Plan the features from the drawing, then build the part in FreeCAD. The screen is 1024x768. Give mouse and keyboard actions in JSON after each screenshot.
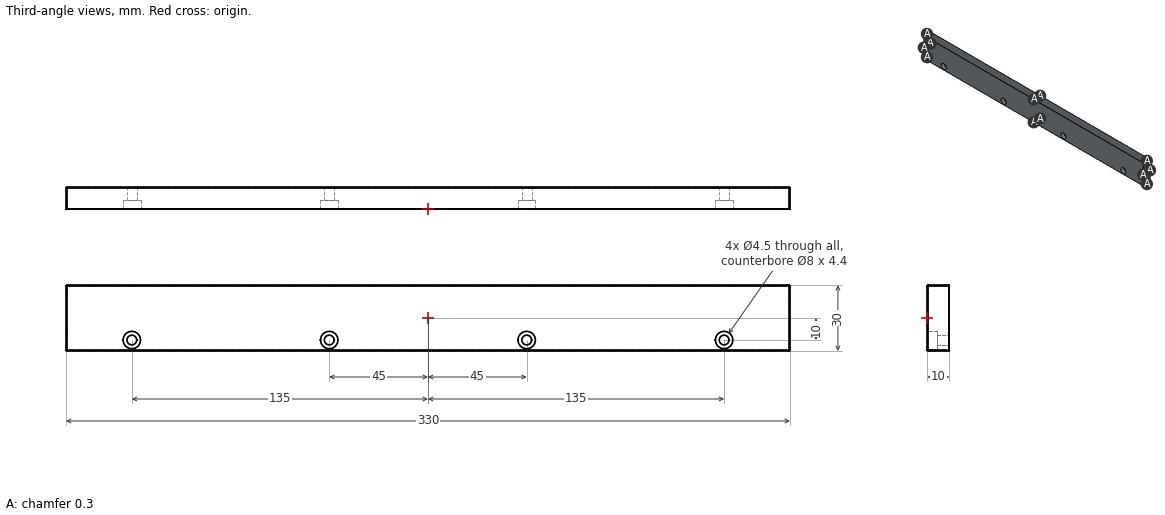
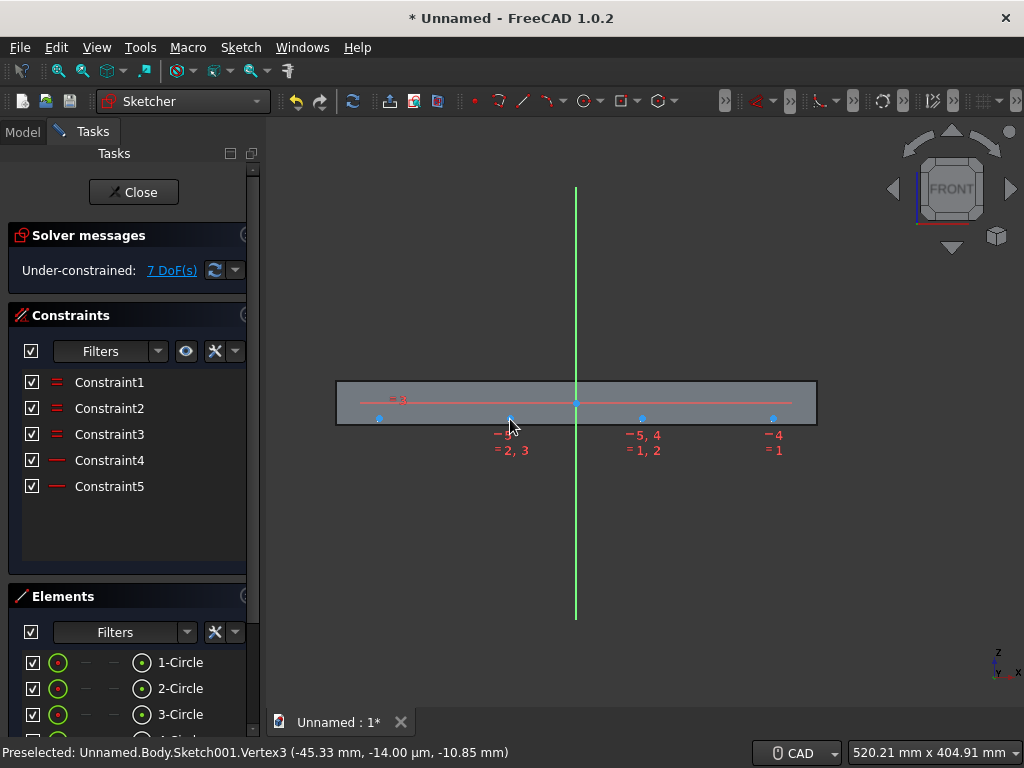
{"action": "left_click", "coordinate": [510, 419]}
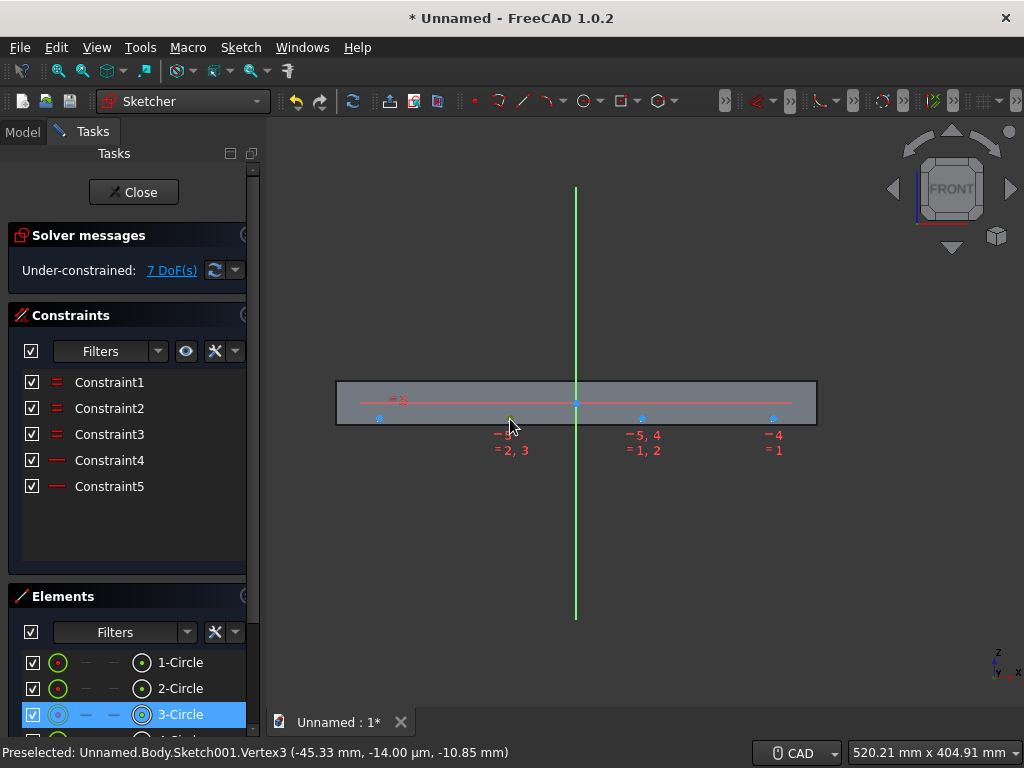
{"action": "left_click", "coordinate": [379, 419]}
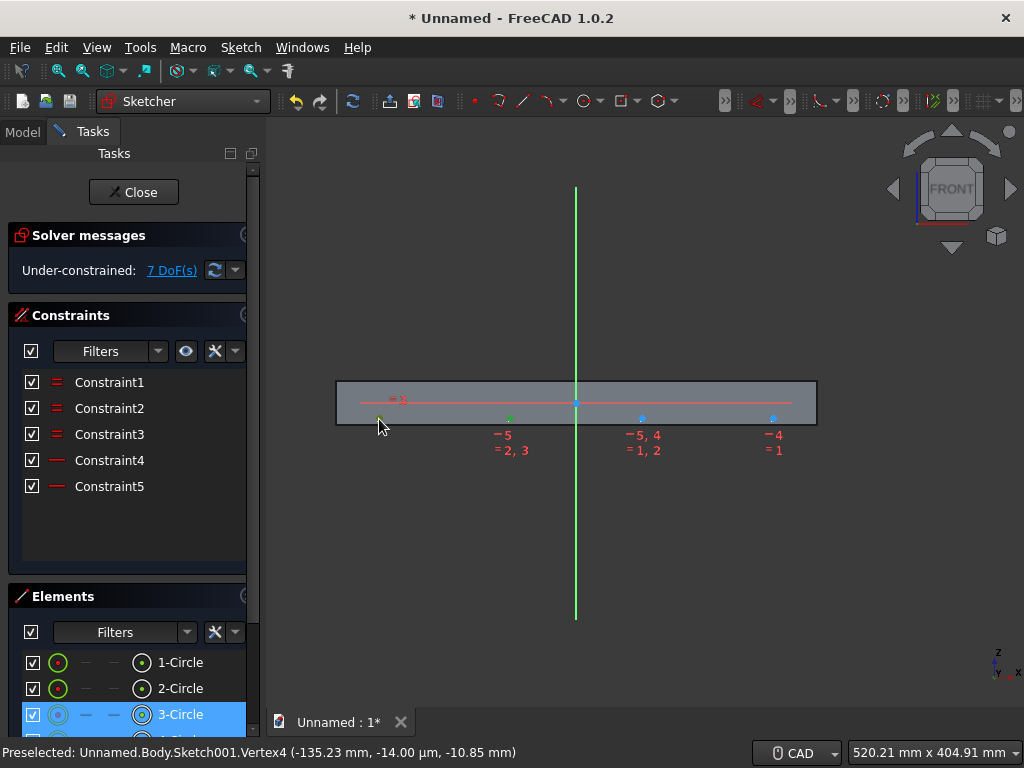
{"action": "key", "text": "h"}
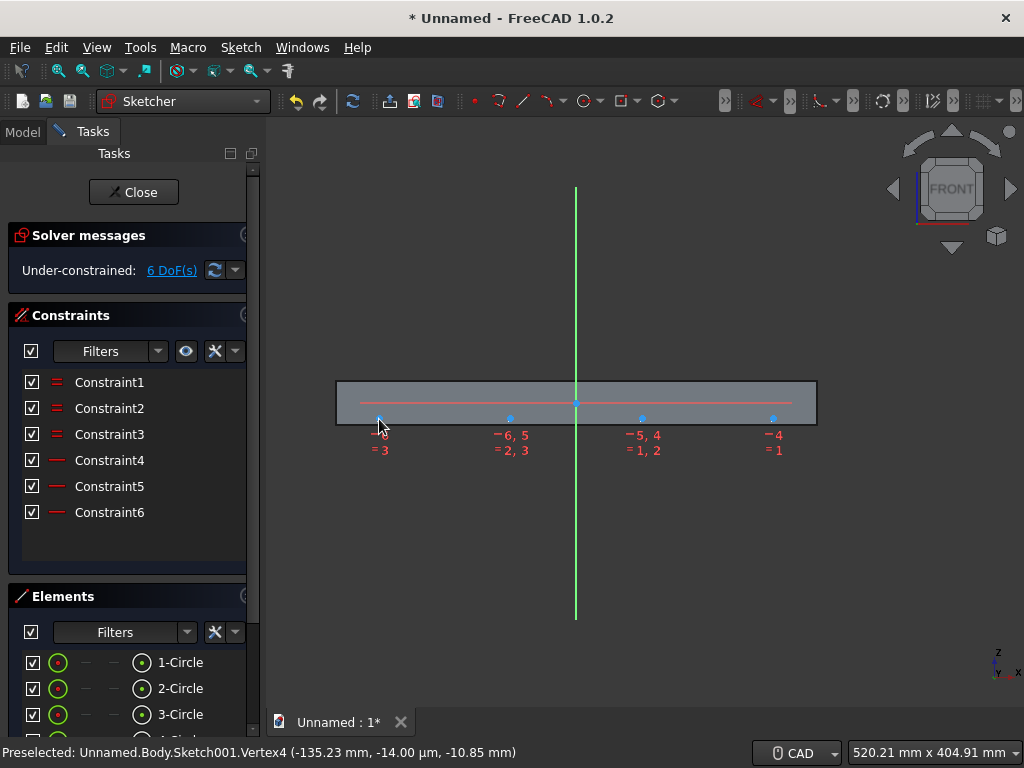
{"action": "key", "text": "d"}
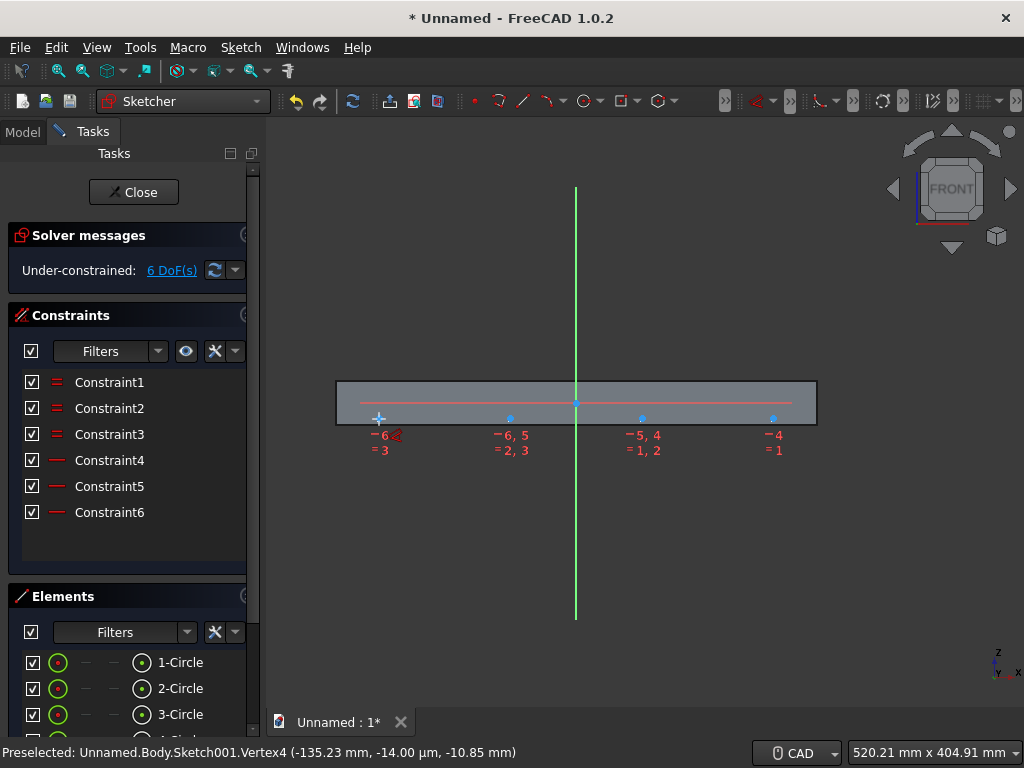
{"action": "scroll", "coordinate": [771, 417], "scroll_direction": "up", "scroll_amount": 10}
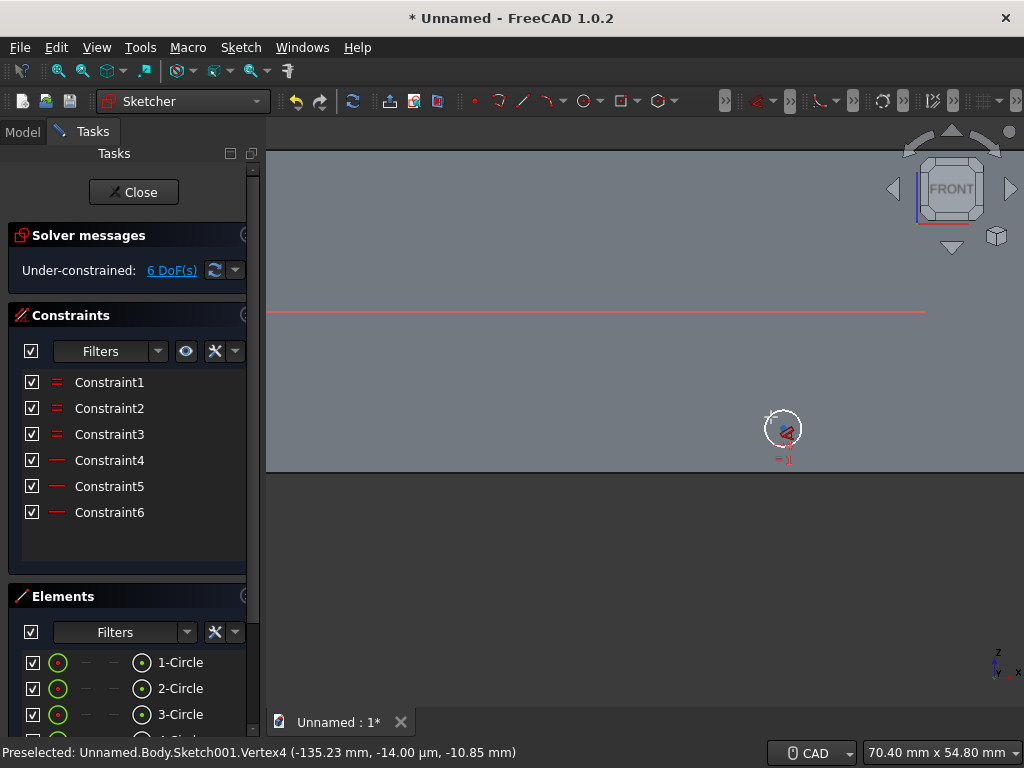
{"action": "left_click", "coordinate": [770, 416]}
{"action": "left_click", "coordinate": [747, 394]}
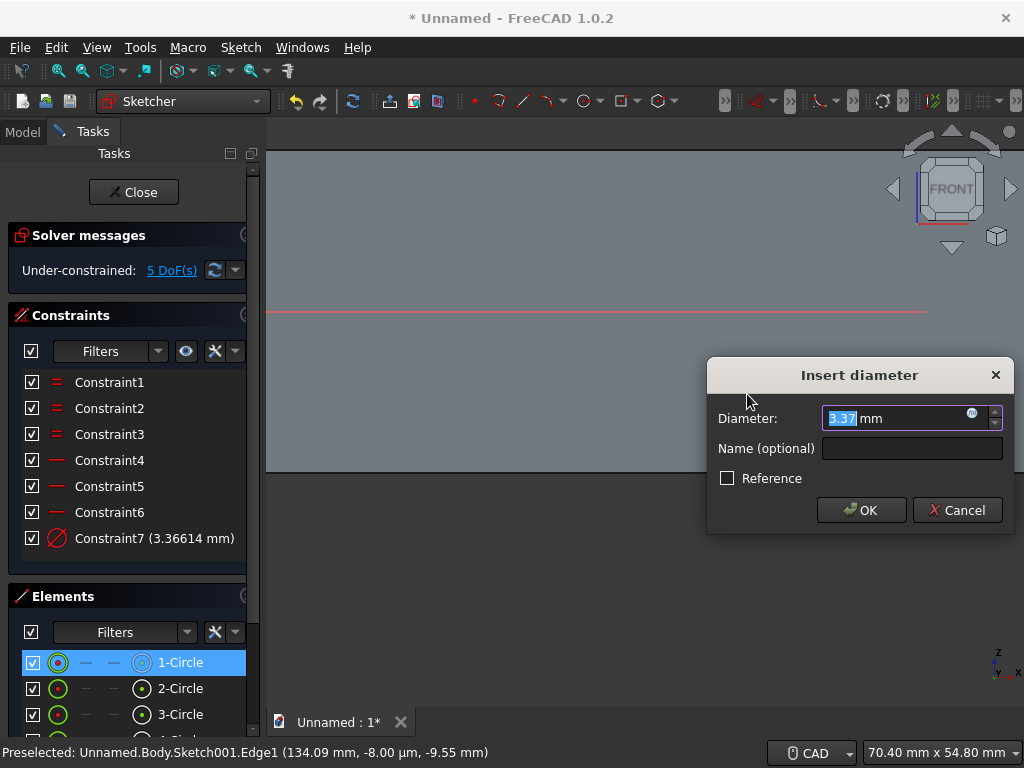
{"action": "type", "text": "4.5"}
{"action": "key", "text": "Return"}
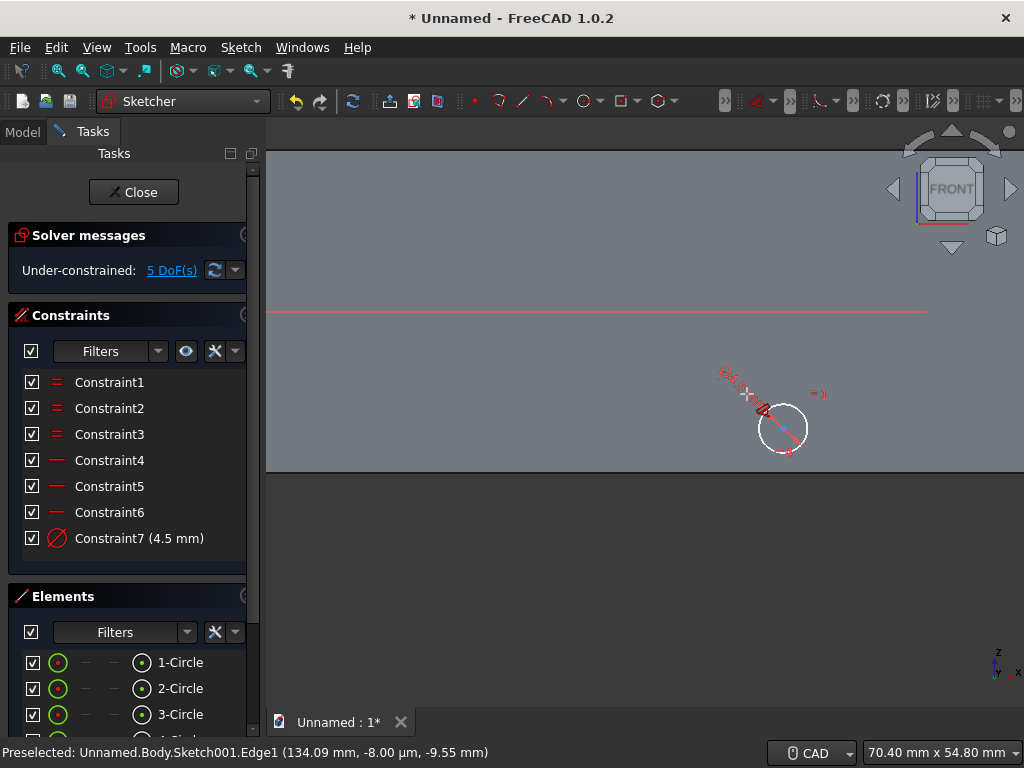
{"action": "left_click", "coordinate": [783, 429]}
{"action": "left_click", "coordinate": [817, 370]}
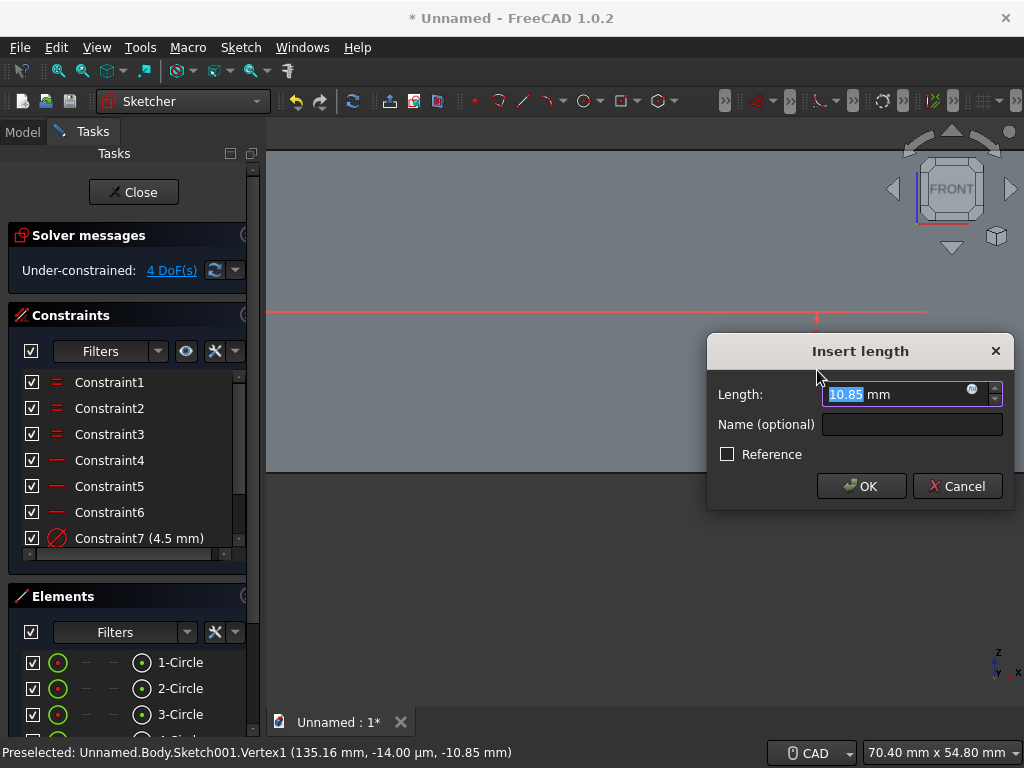
{"action": "type", "text": "10"}
{"action": "key", "text": "Return"}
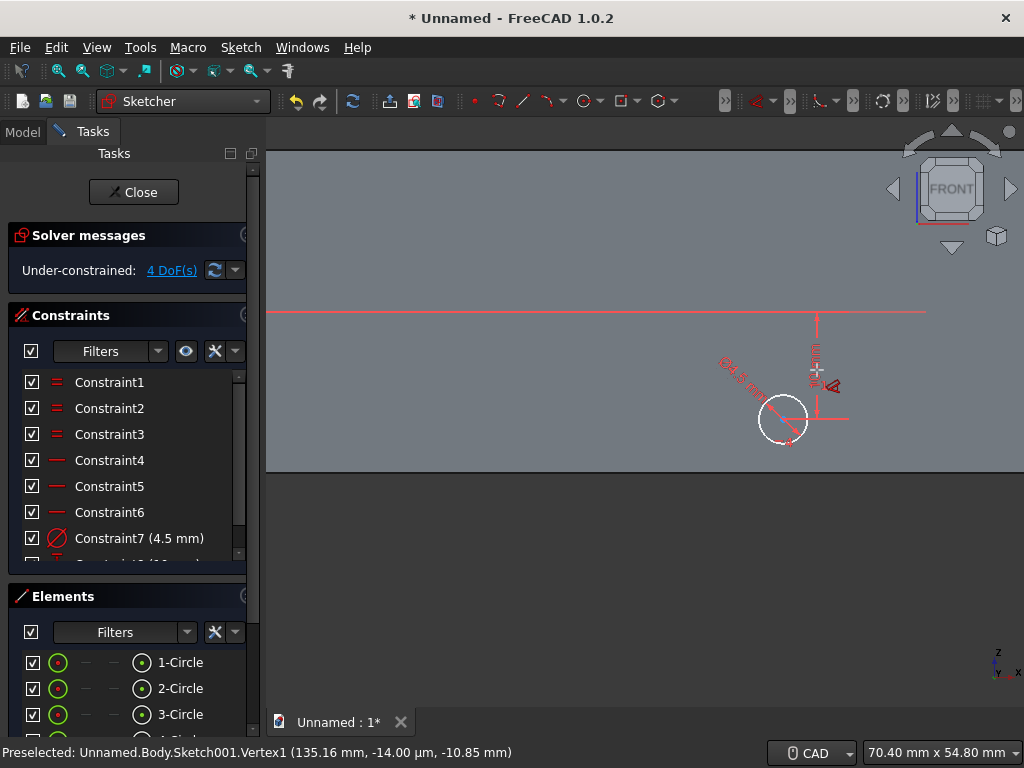
{"action": "scroll", "coordinate": [772, 417], "scroll_direction": "down", "scroll_amount": 10}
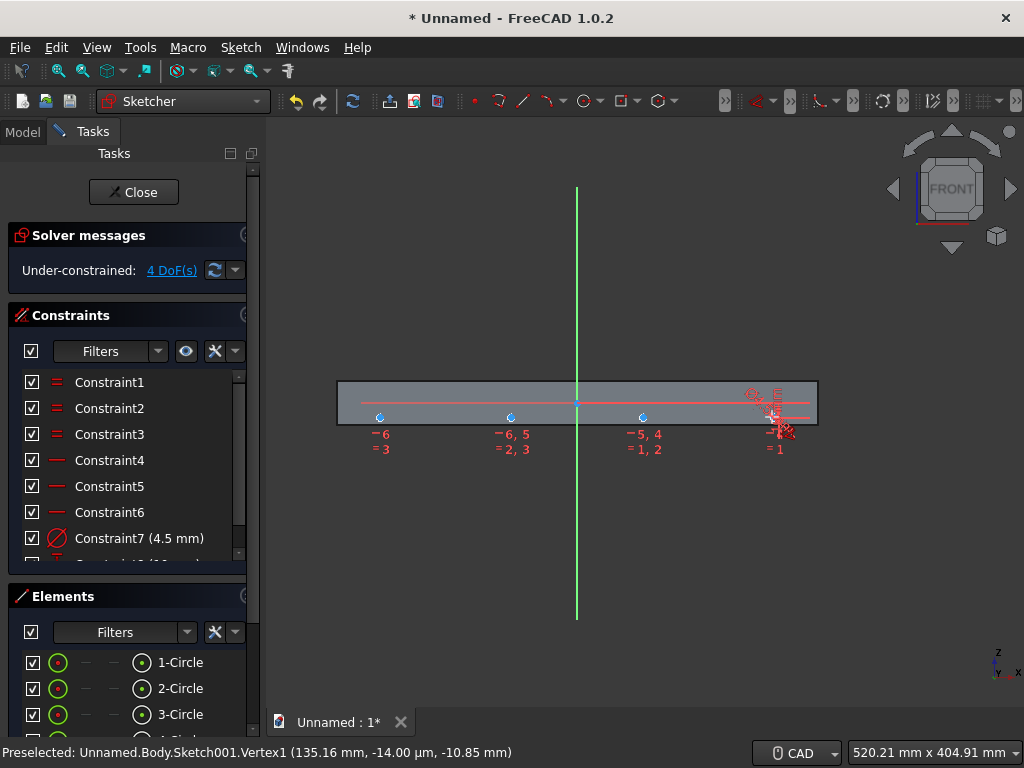
{"action": "left_click", "coordinate": [643, 418]}
{"action": "left_click", "coordinate": [610, 369]}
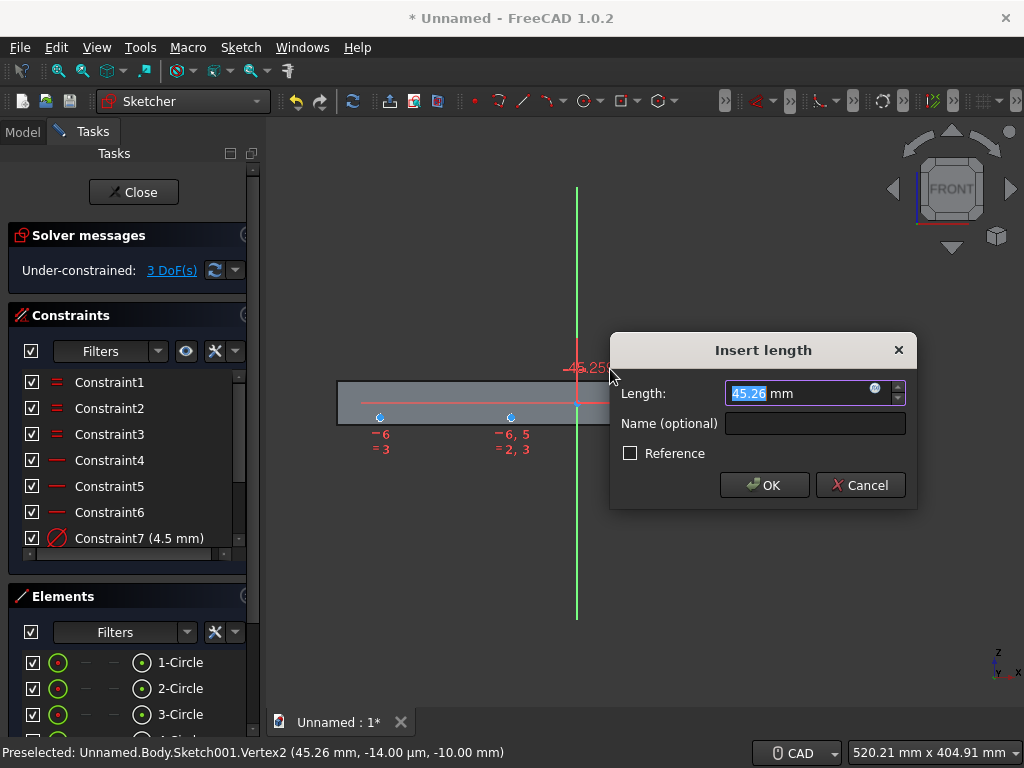
{"action": "type", "text": "45"}
{"action": "key", "text": "Return"}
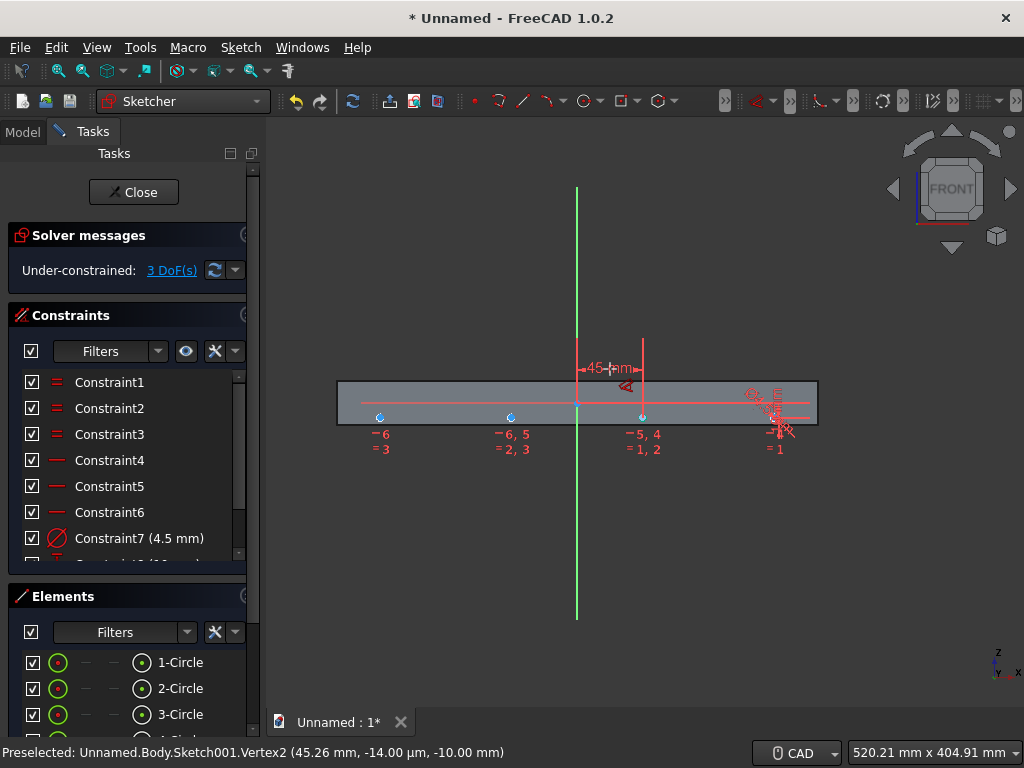
{"action": "left_click", "coordinate": [511, 418]}
{"action": "left_click", "coordinate": [529, 369]}